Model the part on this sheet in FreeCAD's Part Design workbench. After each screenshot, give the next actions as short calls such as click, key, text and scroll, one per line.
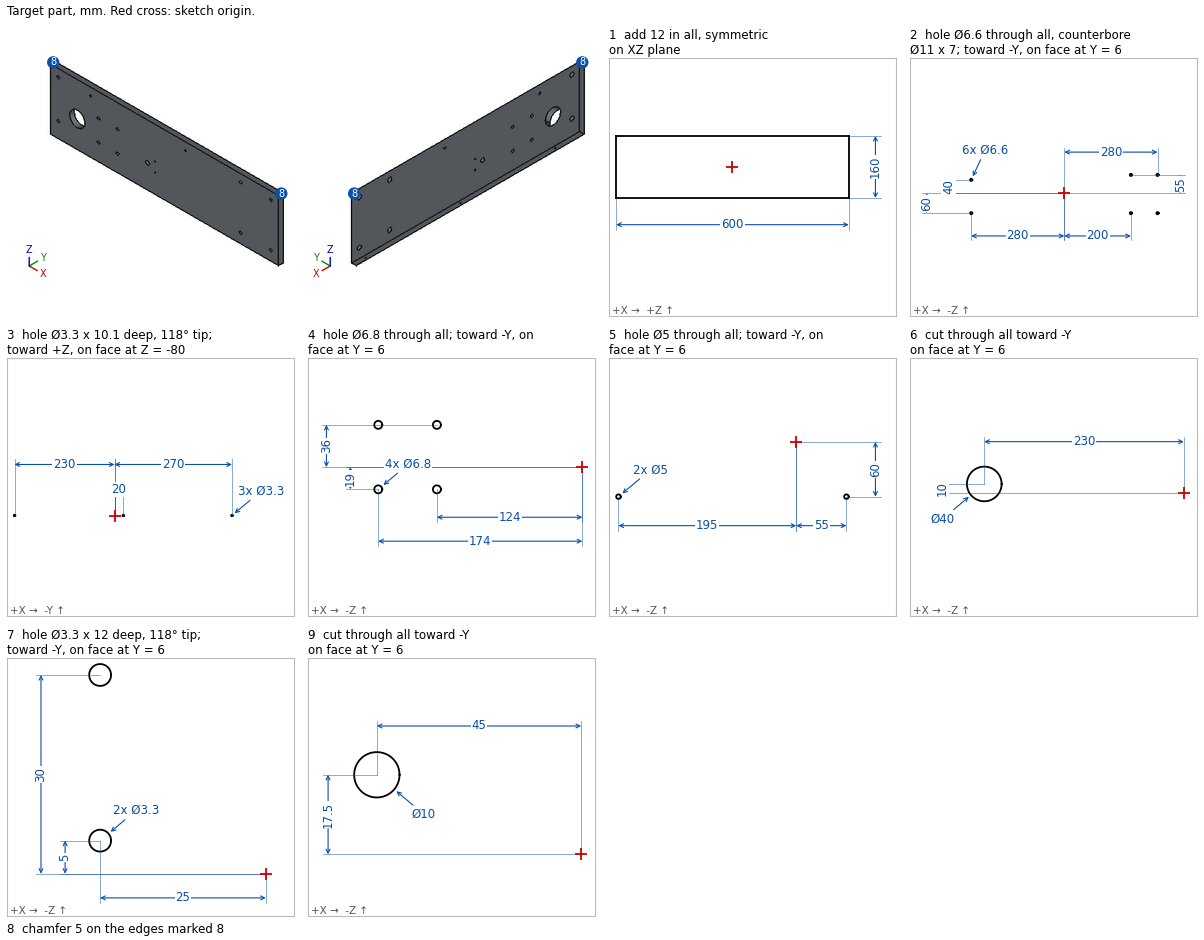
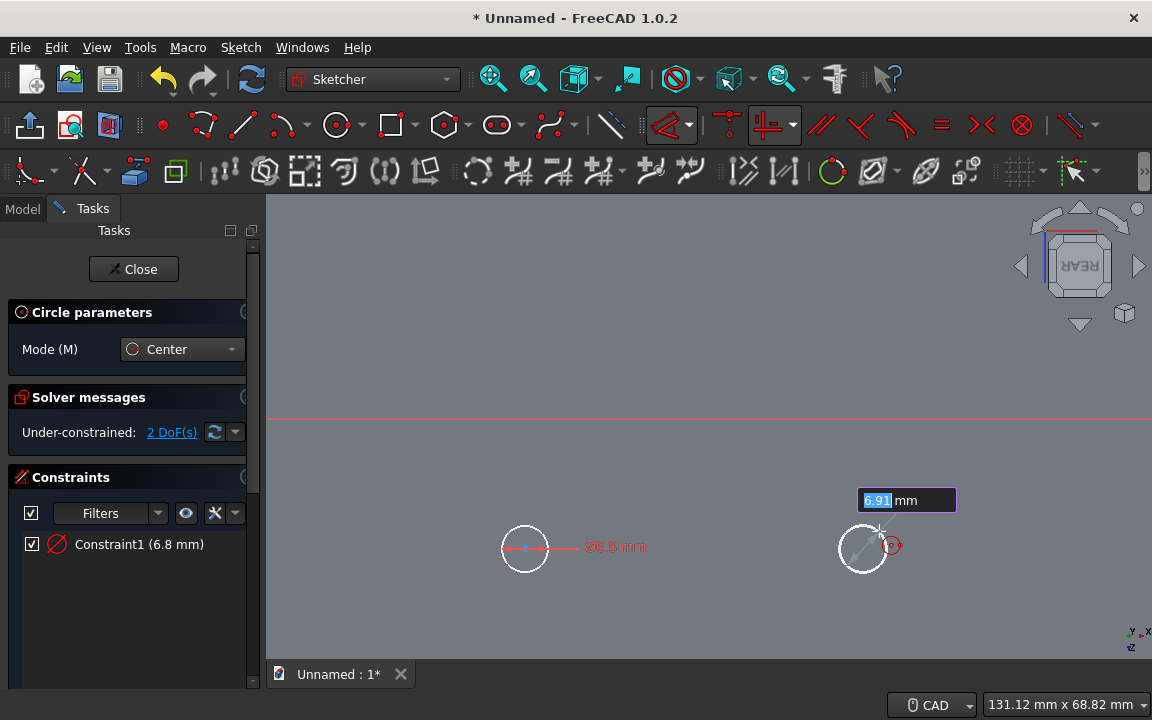
text(6.8)
key(Return)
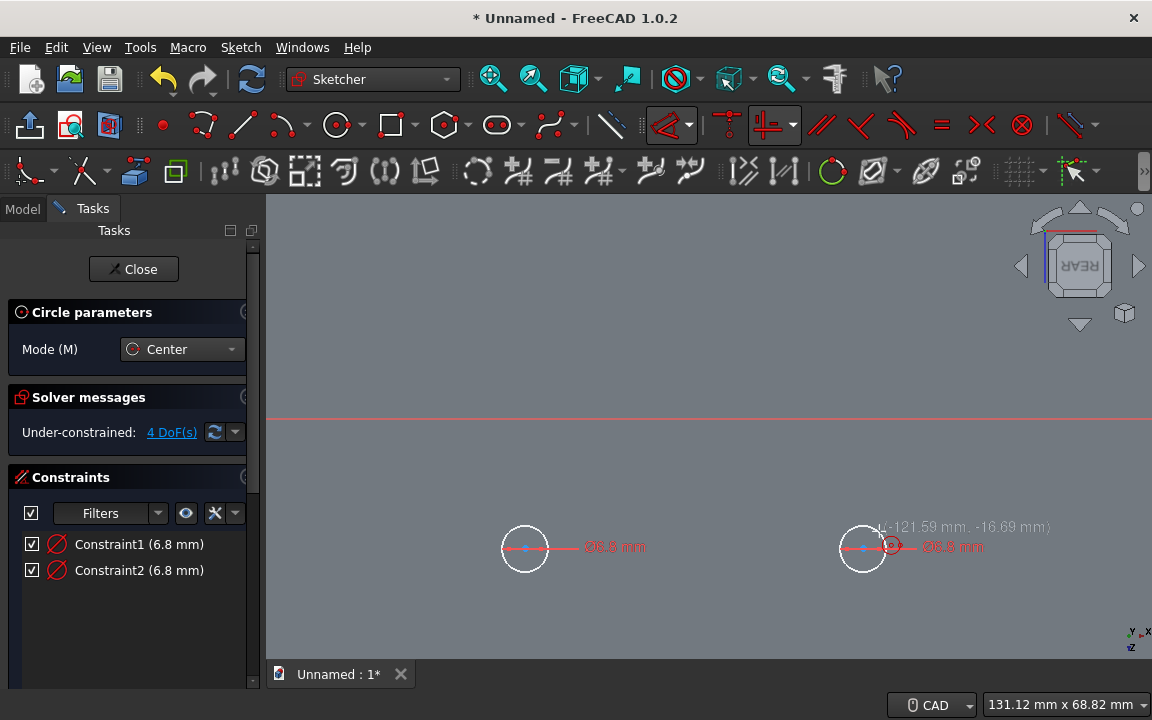
scroll(532, 558, down, 2)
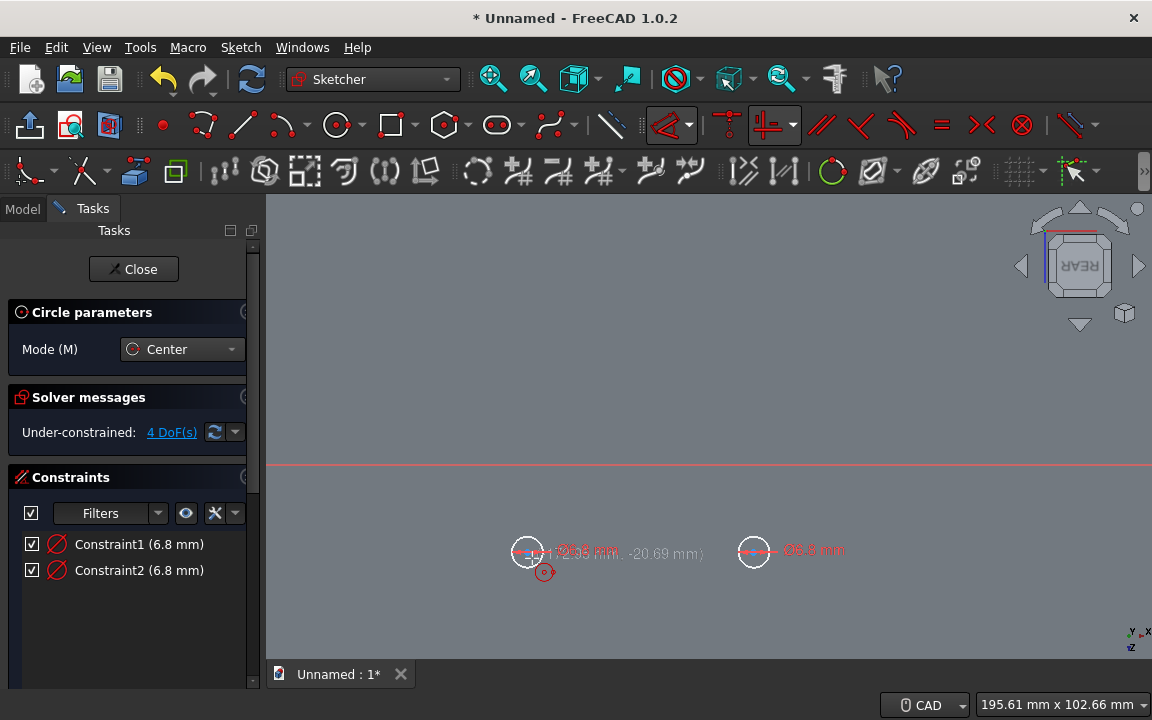
scroll(754, 302, up, 2)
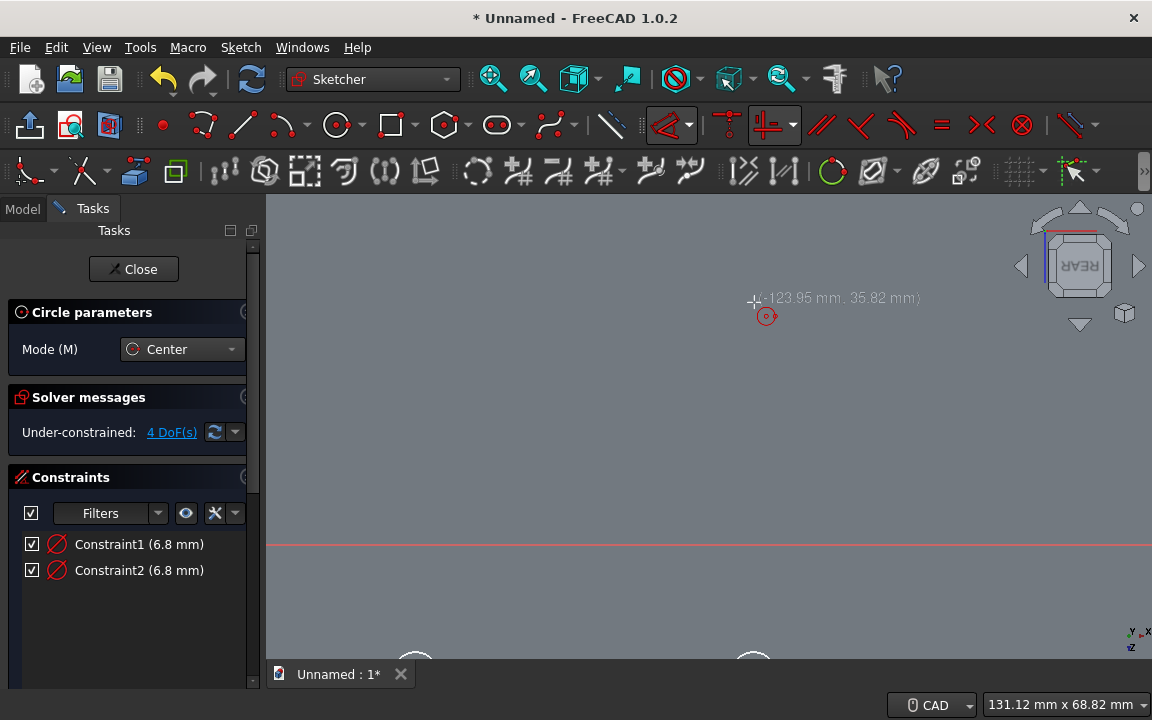
click(753, 302)
move(770, 286)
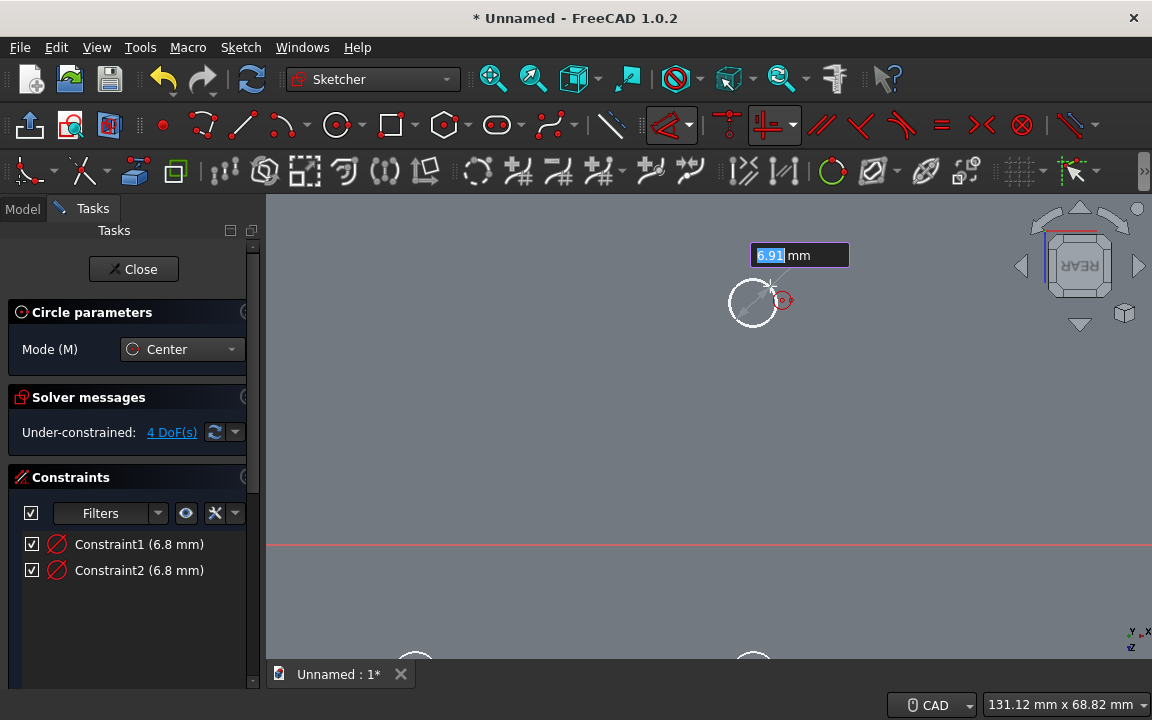
text(6.8)
key(Return)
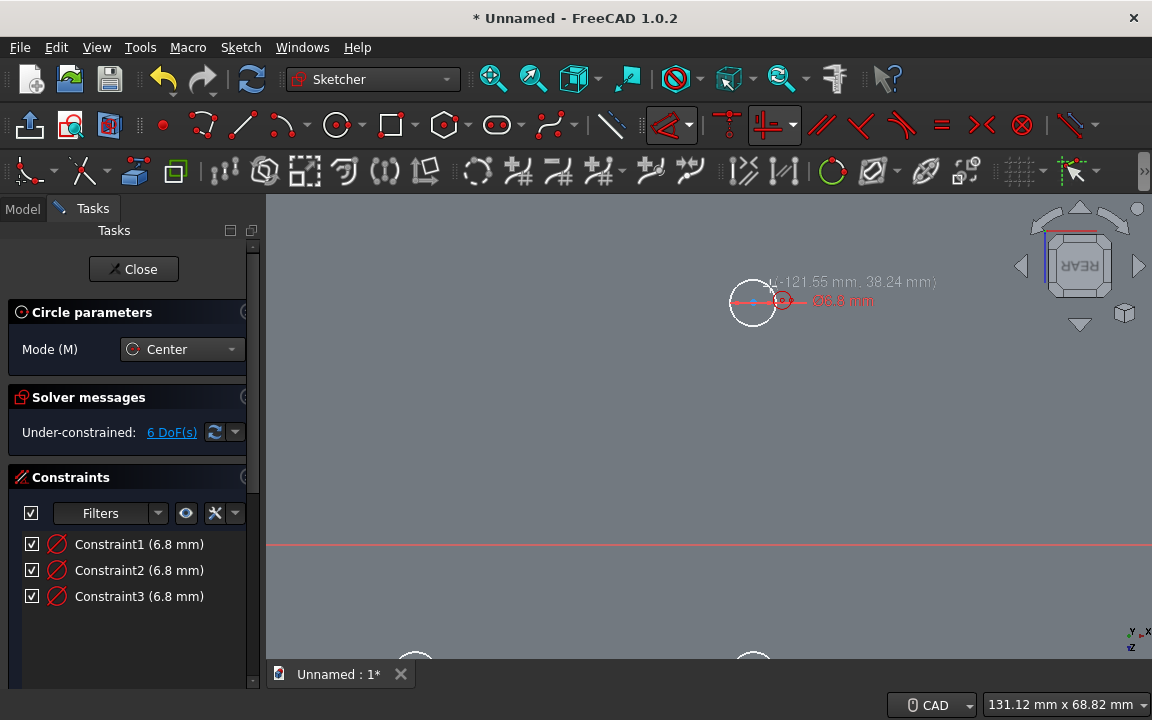
click(416, 302)
move(432, 286)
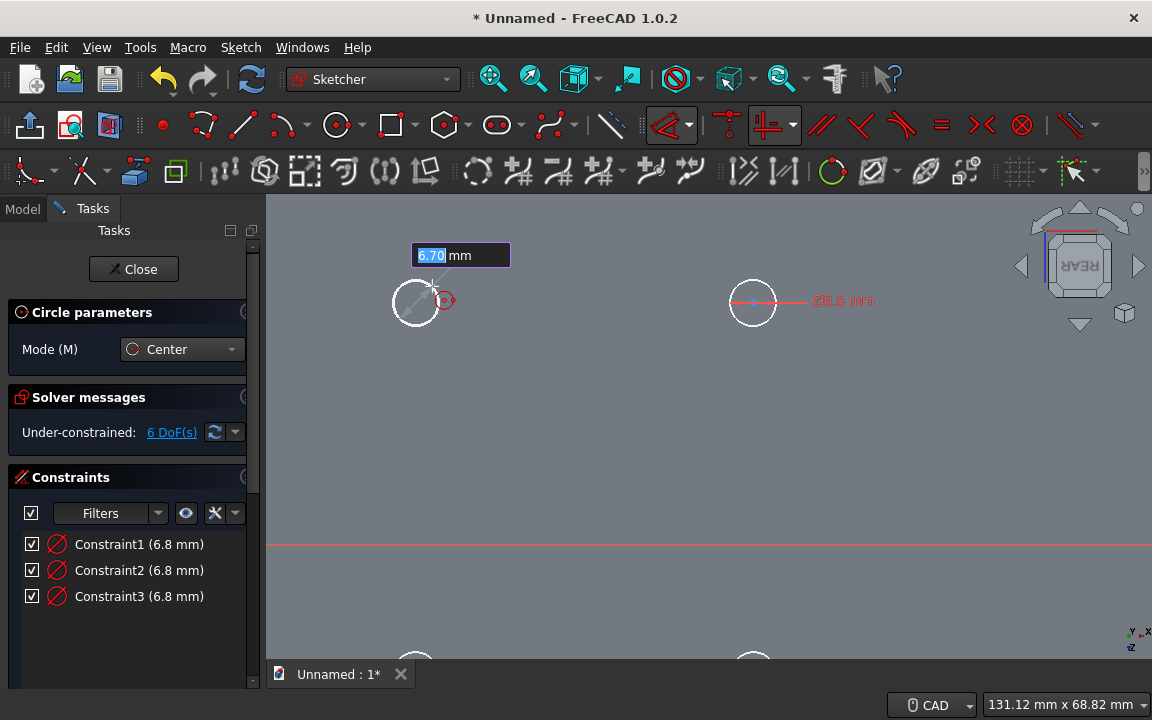
text(6.8)
key(Return)
key(Escape)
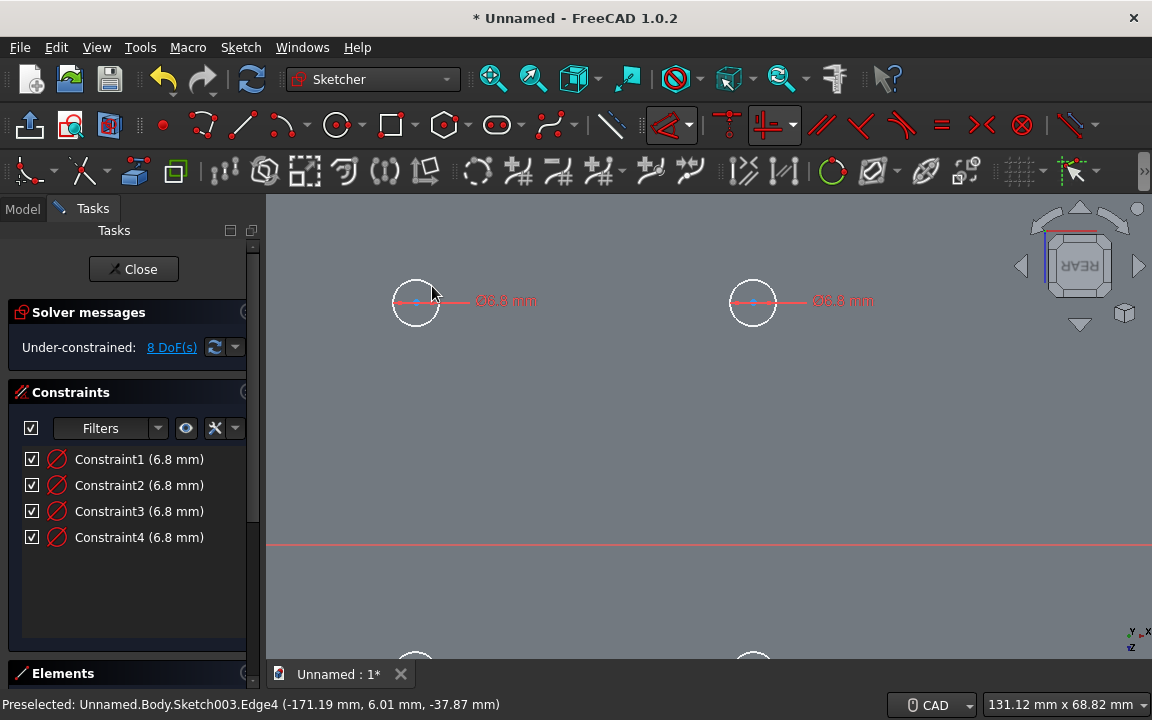
scroll(754, 302, down, 2)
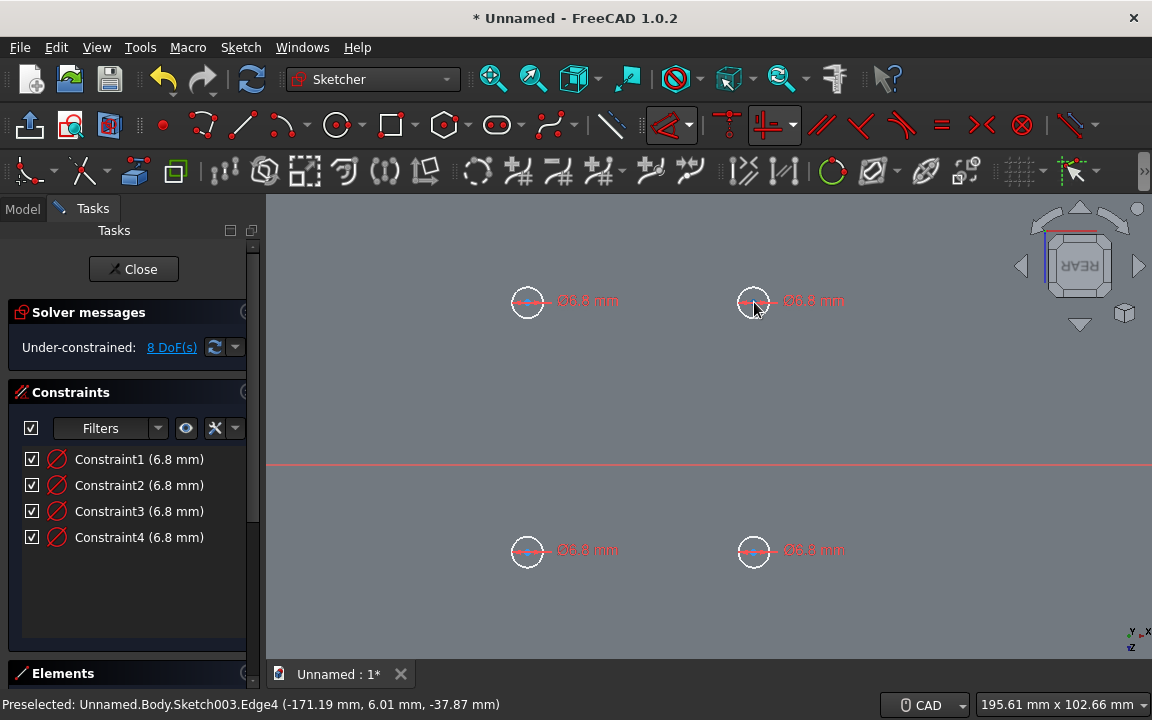
click(527, 552)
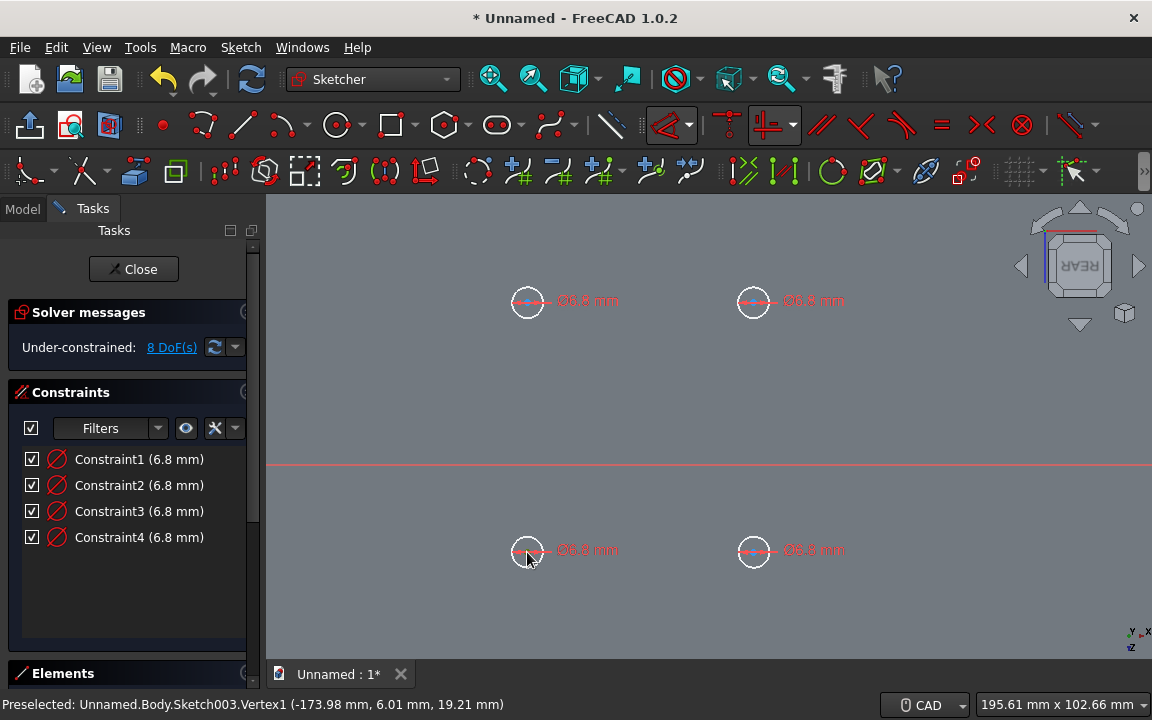
click(754, 552)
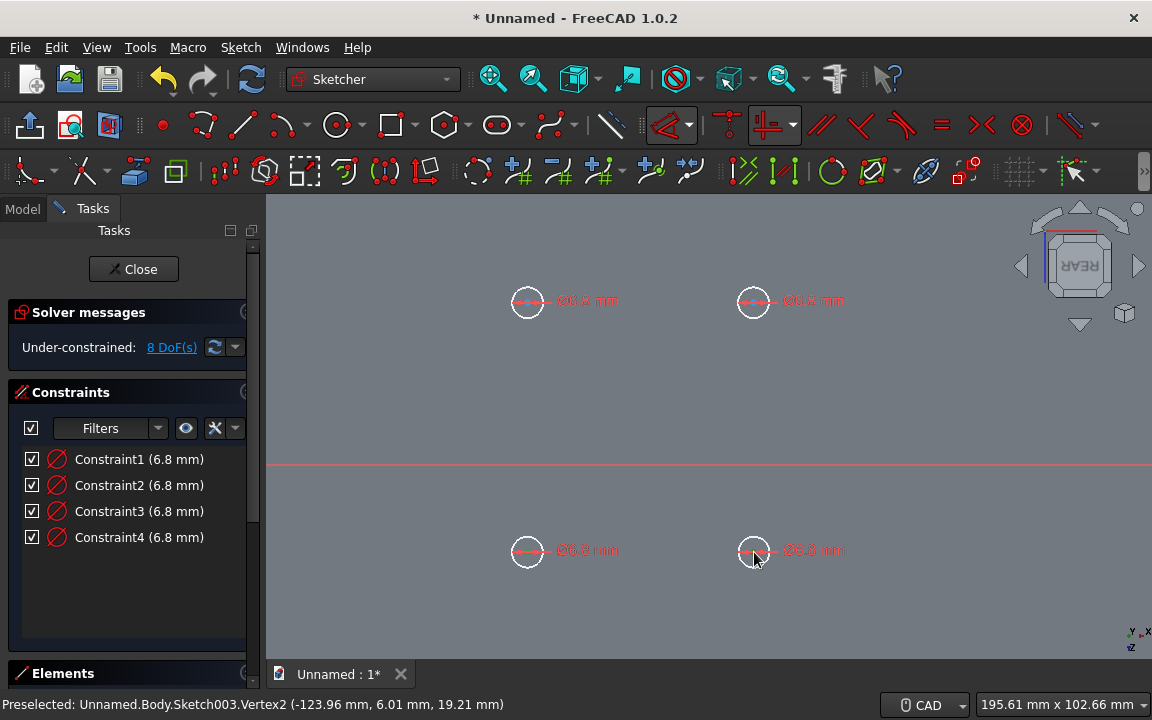
key(h)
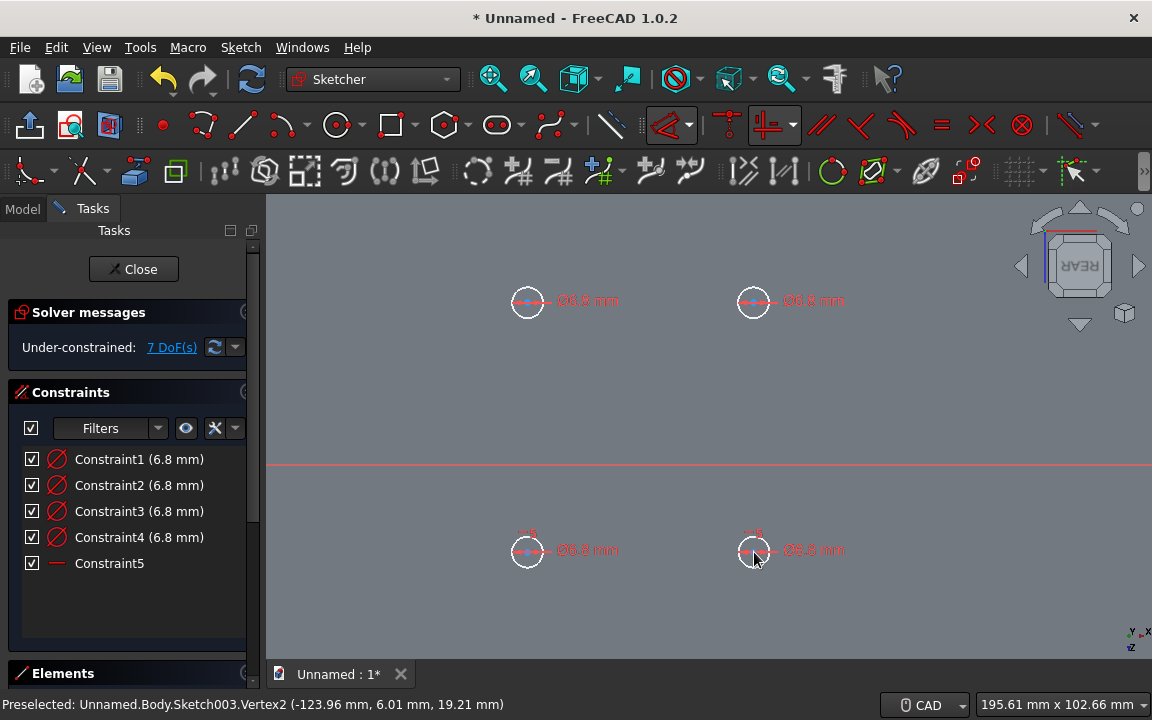
click(754, 552)